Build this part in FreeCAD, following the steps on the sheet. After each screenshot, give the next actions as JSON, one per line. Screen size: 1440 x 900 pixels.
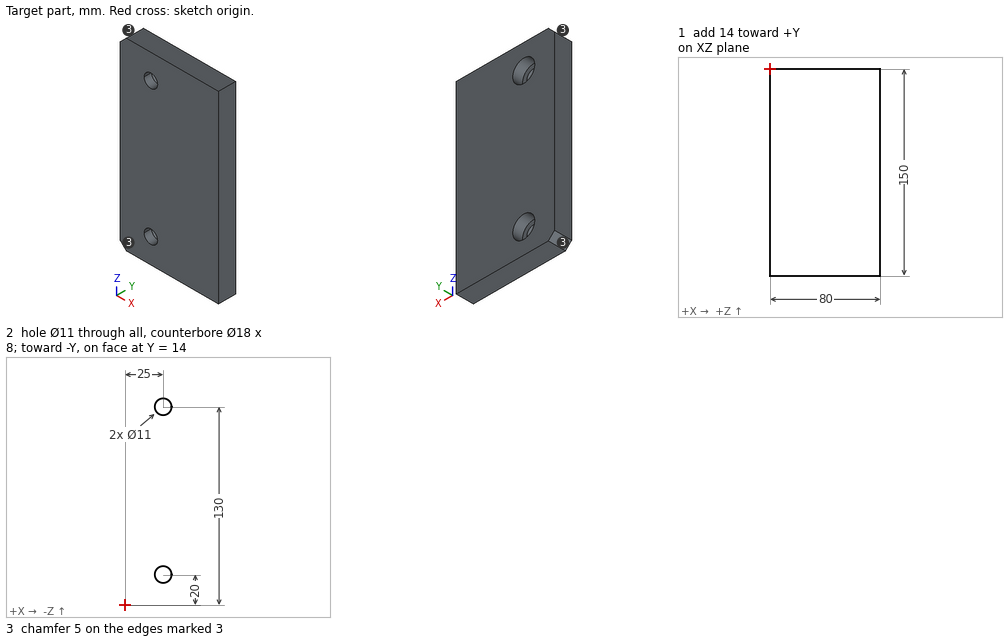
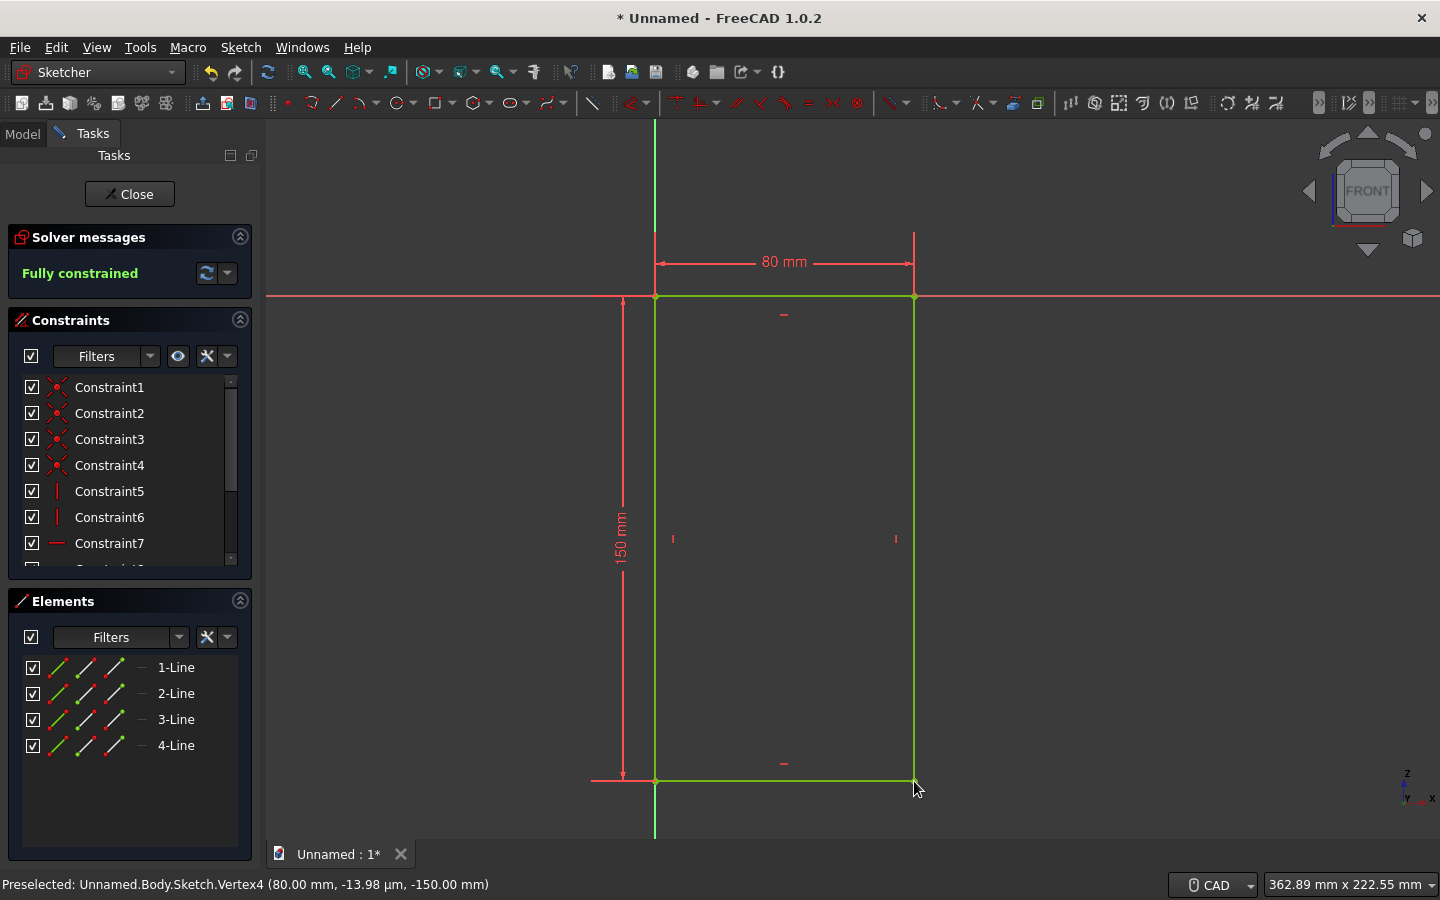
{"action": "left_click", "coordinate": [130, 194]}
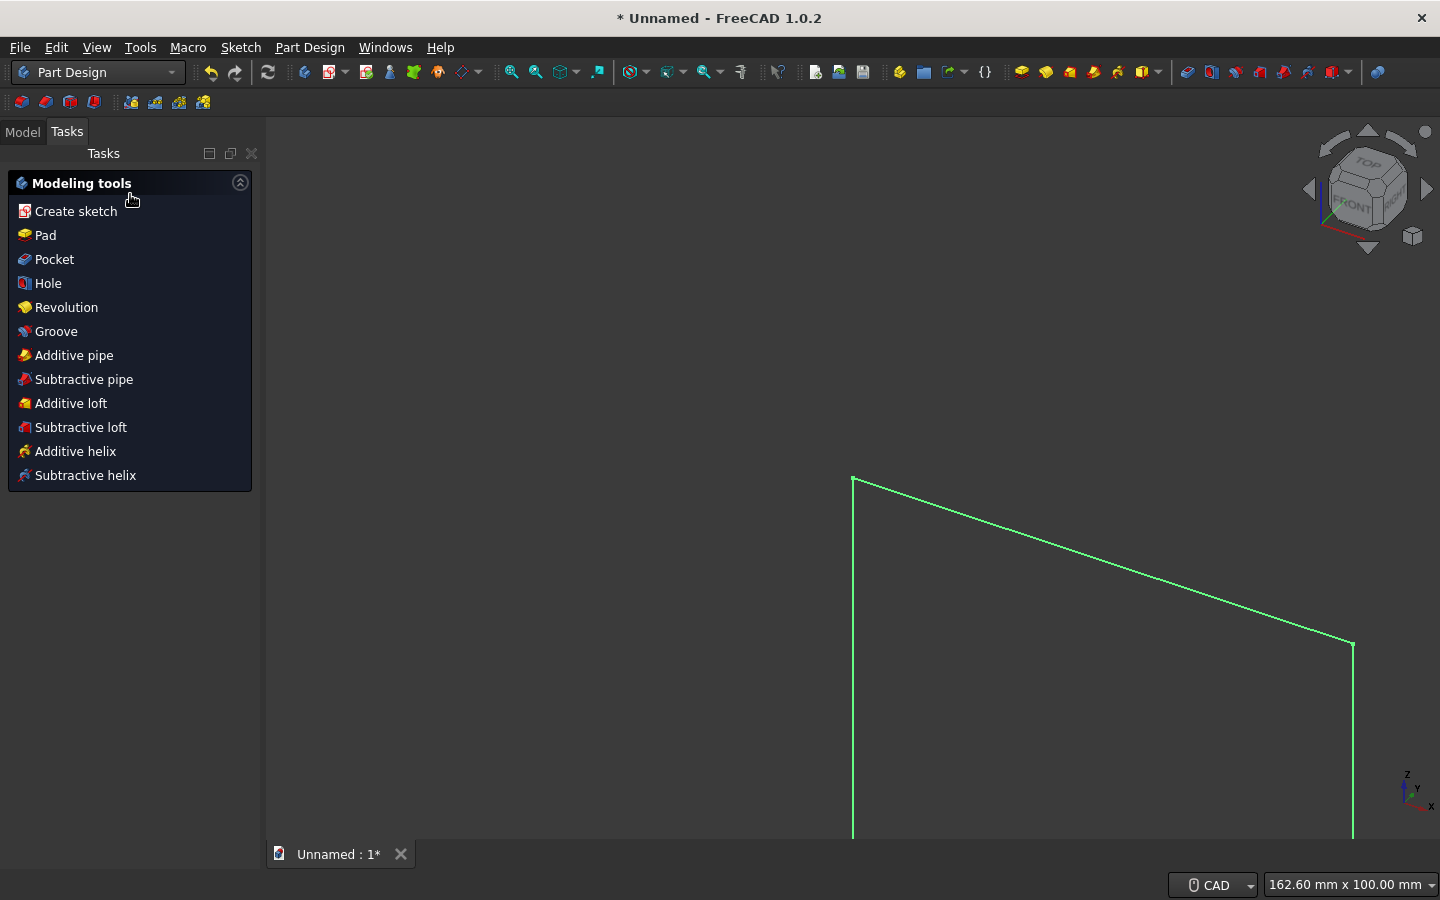
{"action": "left_click", "coordinate": [1022, 72]}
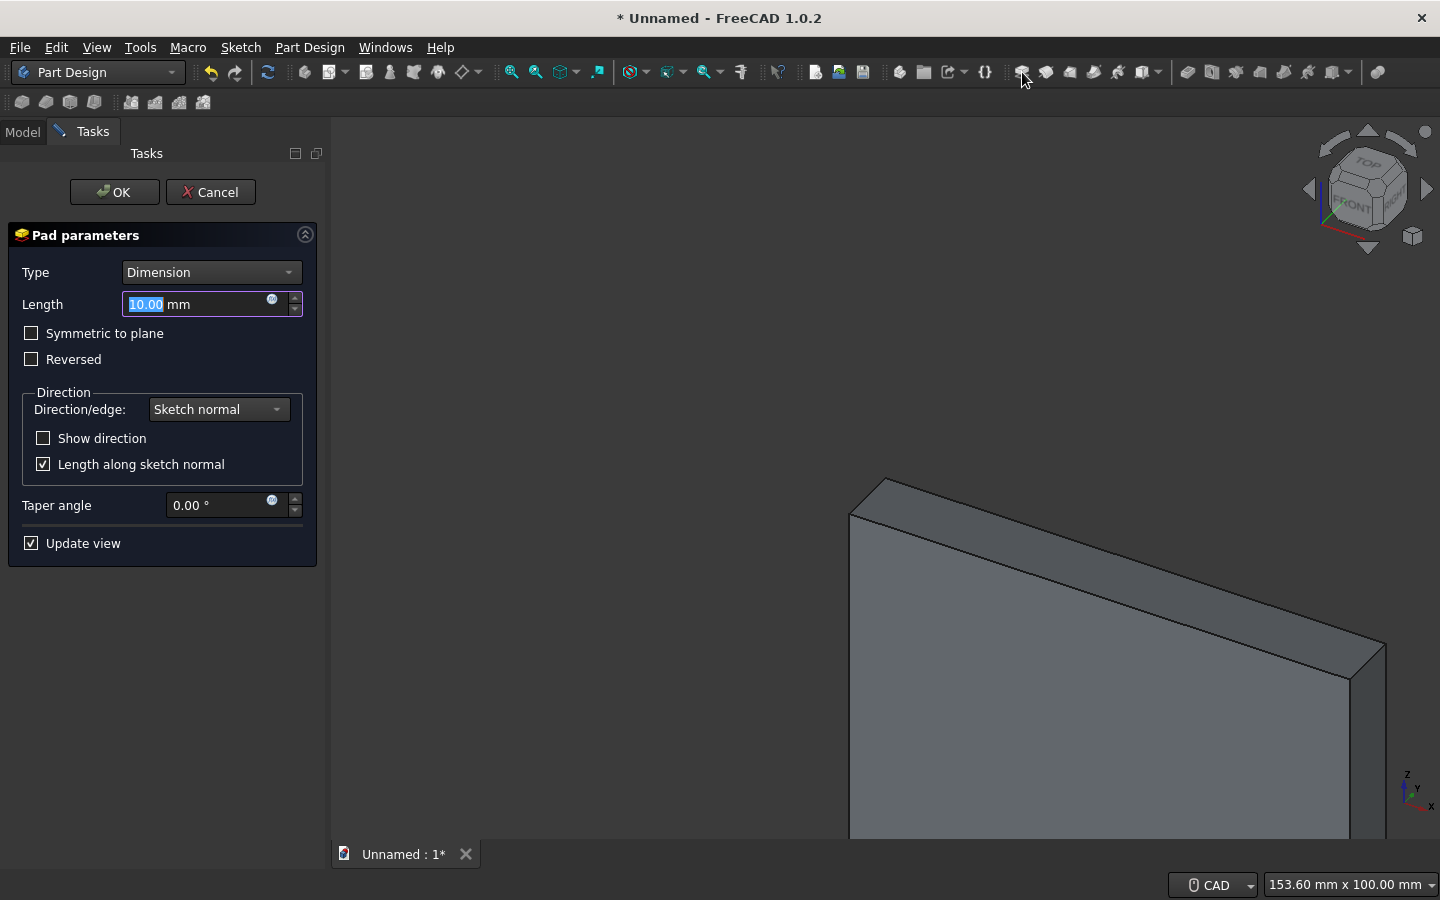
{"action": "type", "text": "14"}
{"action": "key", "text": "Tab"}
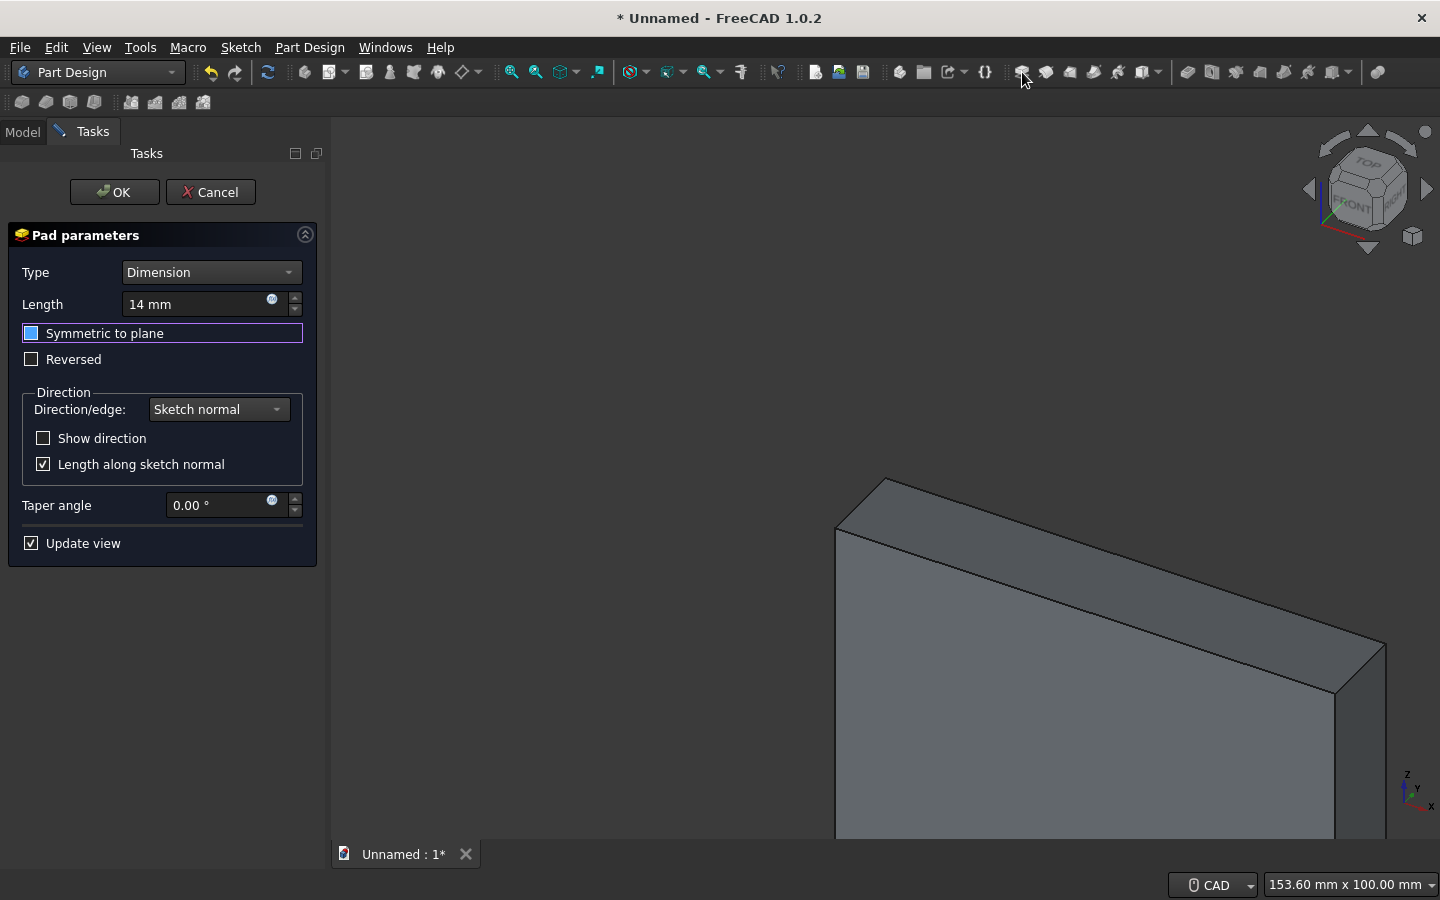
{"action": "left_click", "coordinate": [30, 359]}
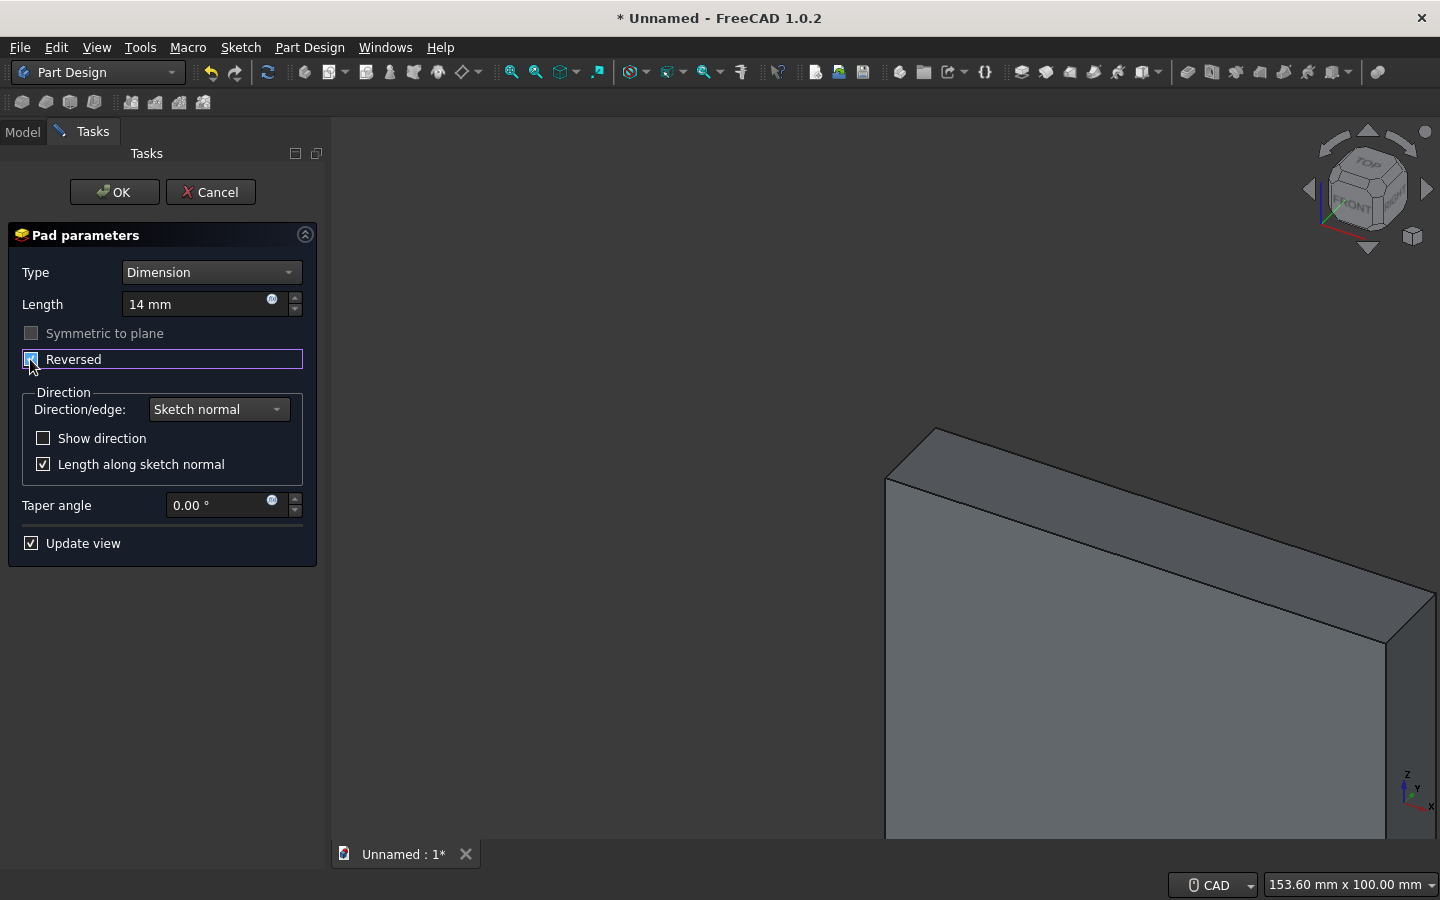
{"action": "left_click", "coordinate": [115, 192]}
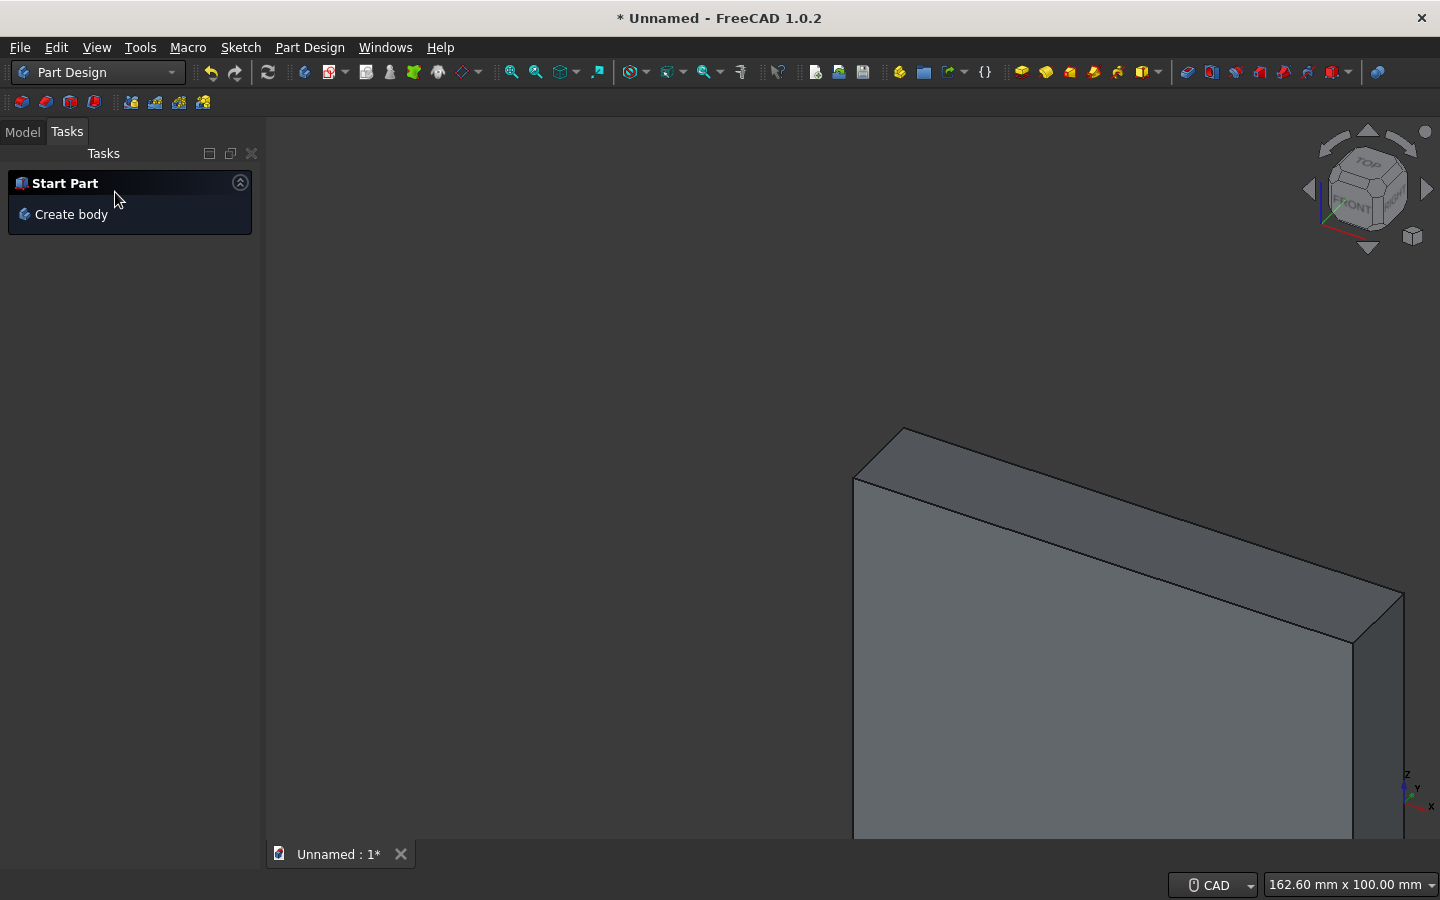
{"action": "left_click", "coordinate": [512, 72]}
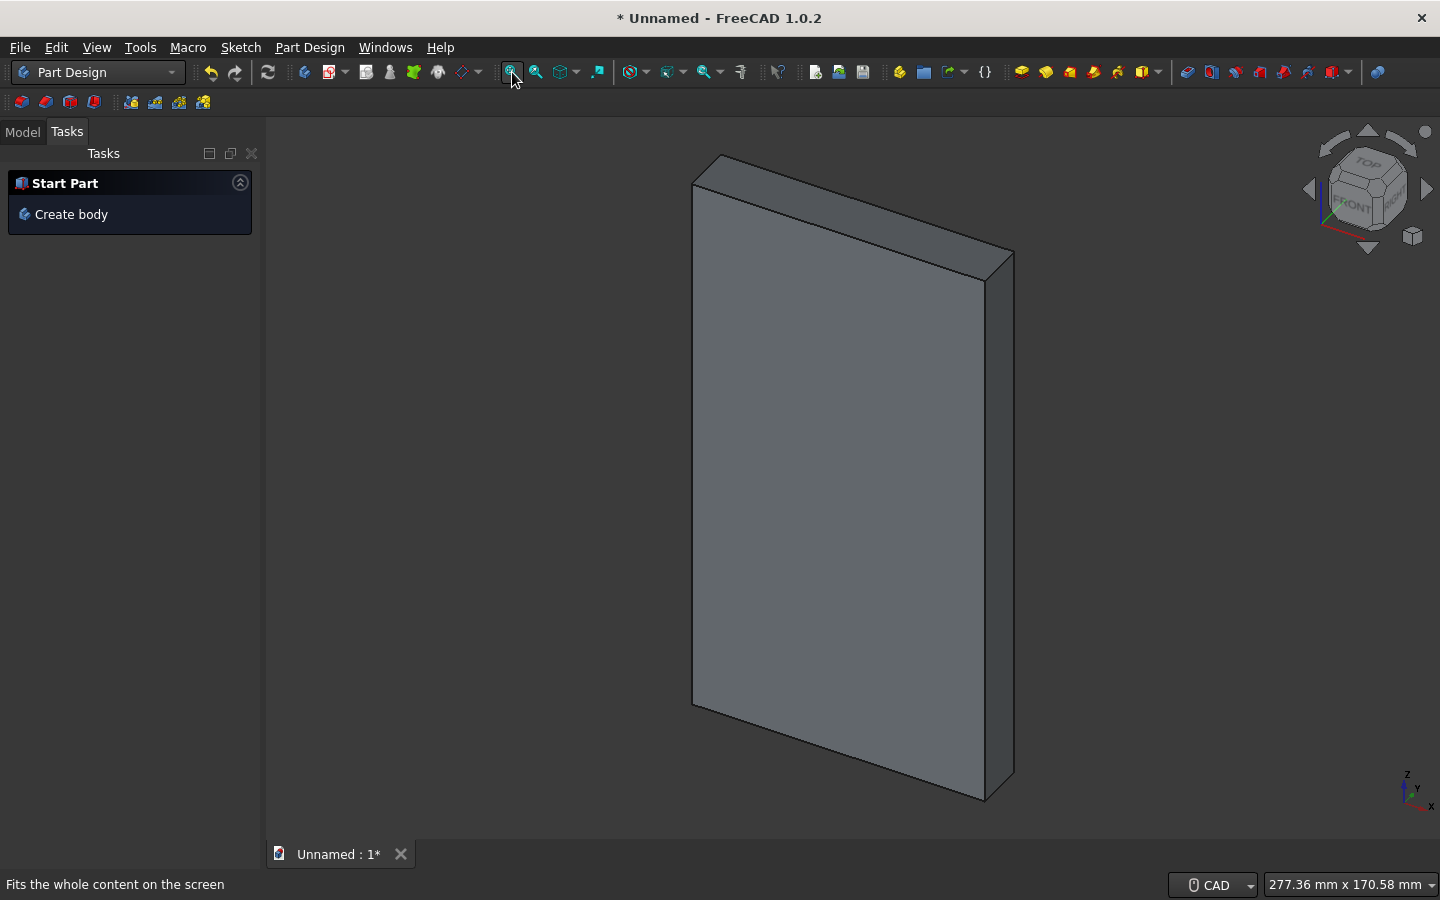
{"action": "key", "text": "4"}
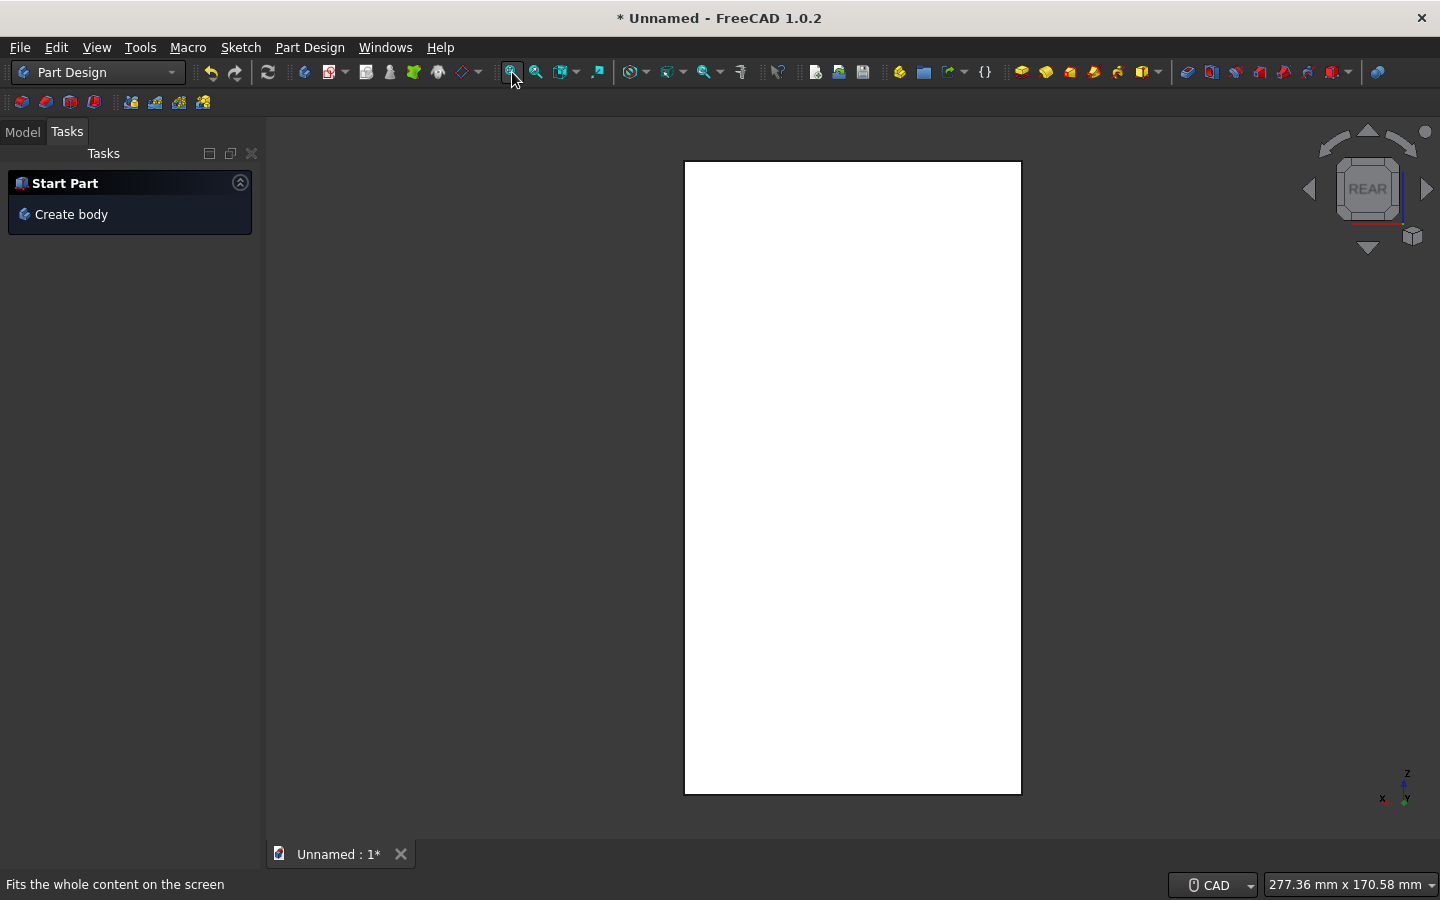
{"action": "left_click", "coordinate": [853, 386]}